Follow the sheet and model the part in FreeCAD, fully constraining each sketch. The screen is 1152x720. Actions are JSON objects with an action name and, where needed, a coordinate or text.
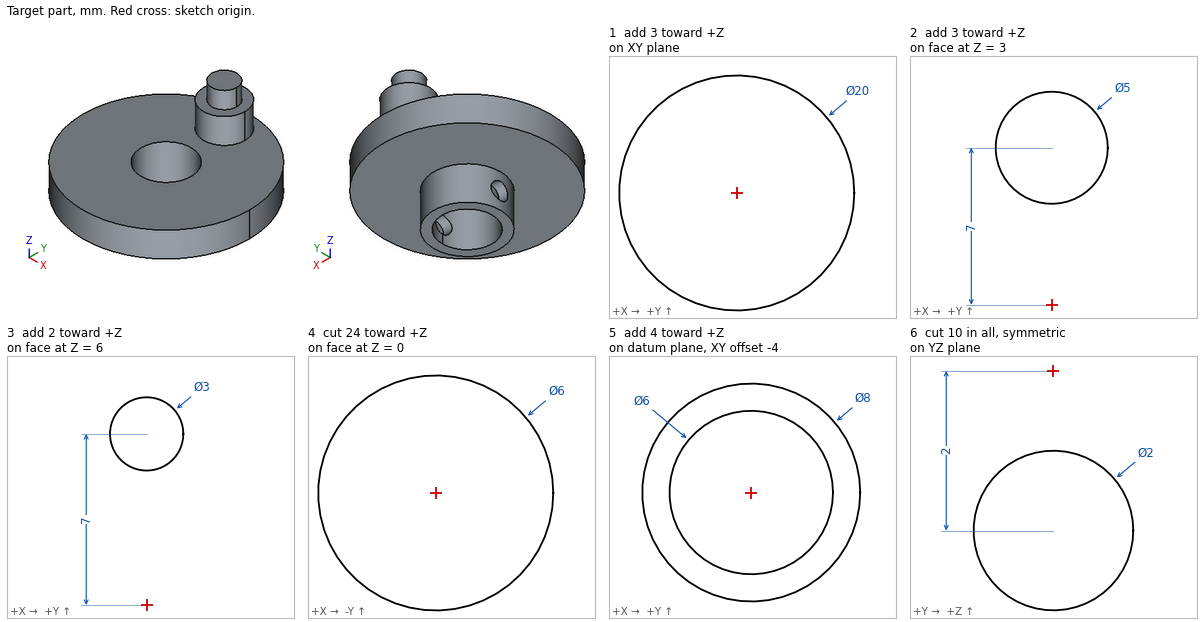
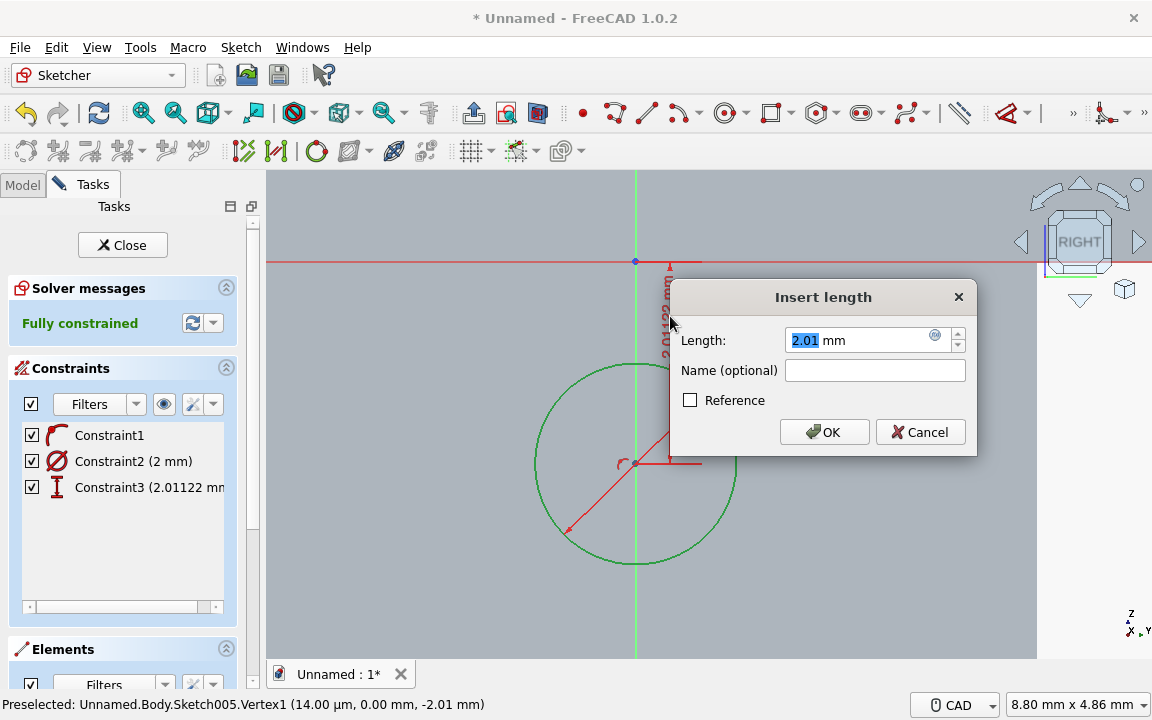
{"action": "type", "text": "2"}
{"action": "key", "text": "Return"}
{"action": "key", "text": "Escape"}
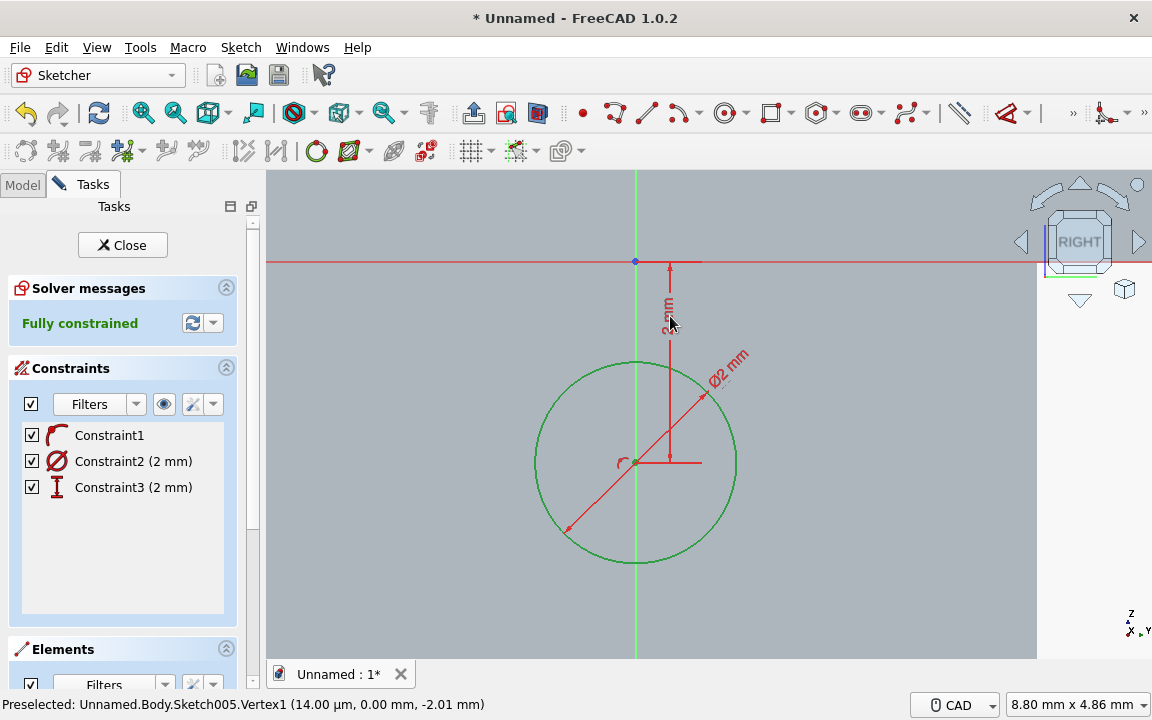
{"action": "left_click", "coordinate": [123, 245]}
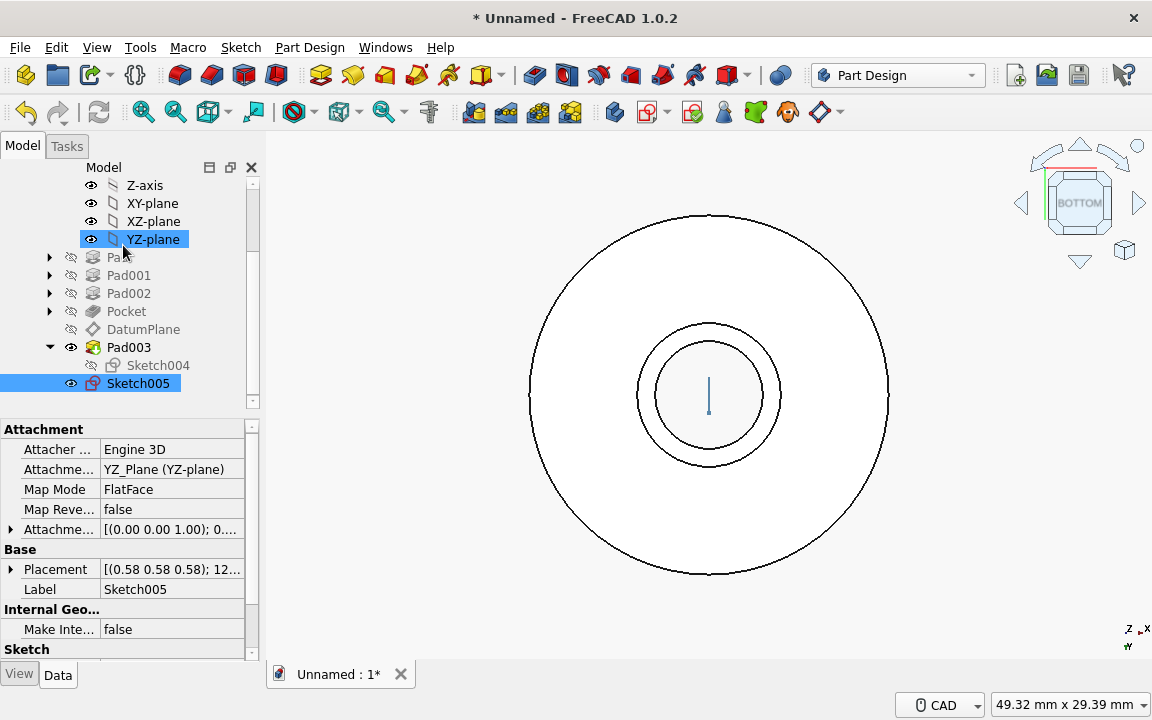
{"action": "left_click", "coordinate": [536, 76]}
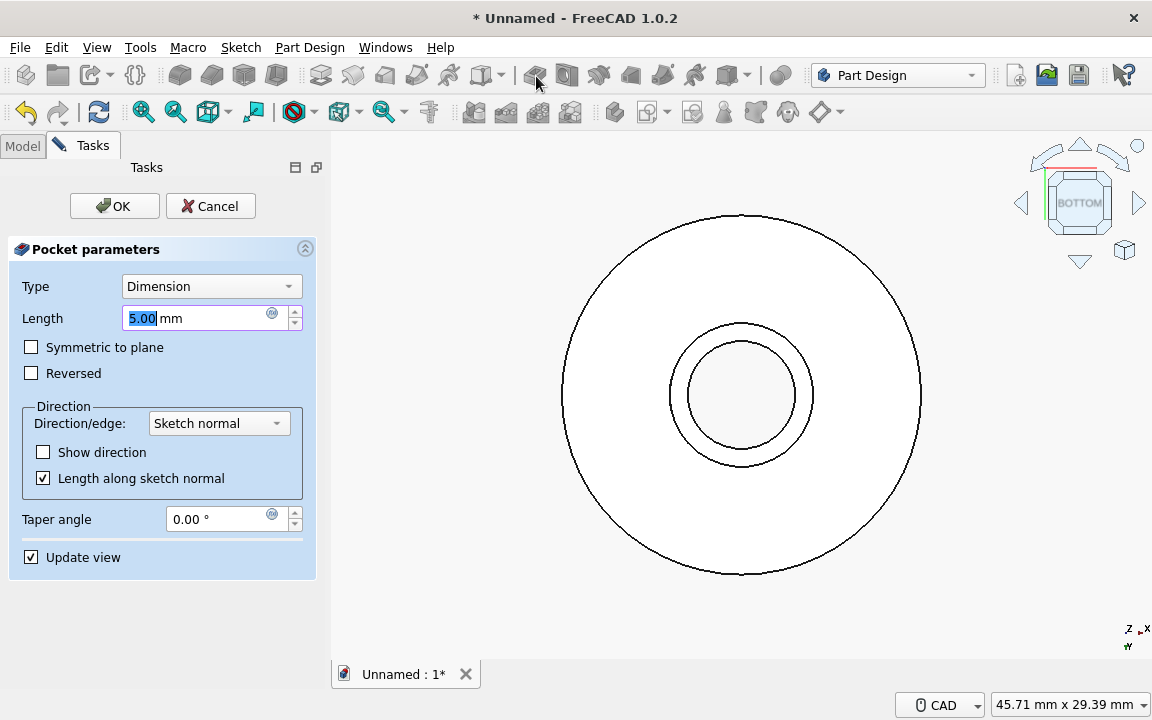
{"action": "type", "text": "10"}
{"action": "key", "text": "Tab"}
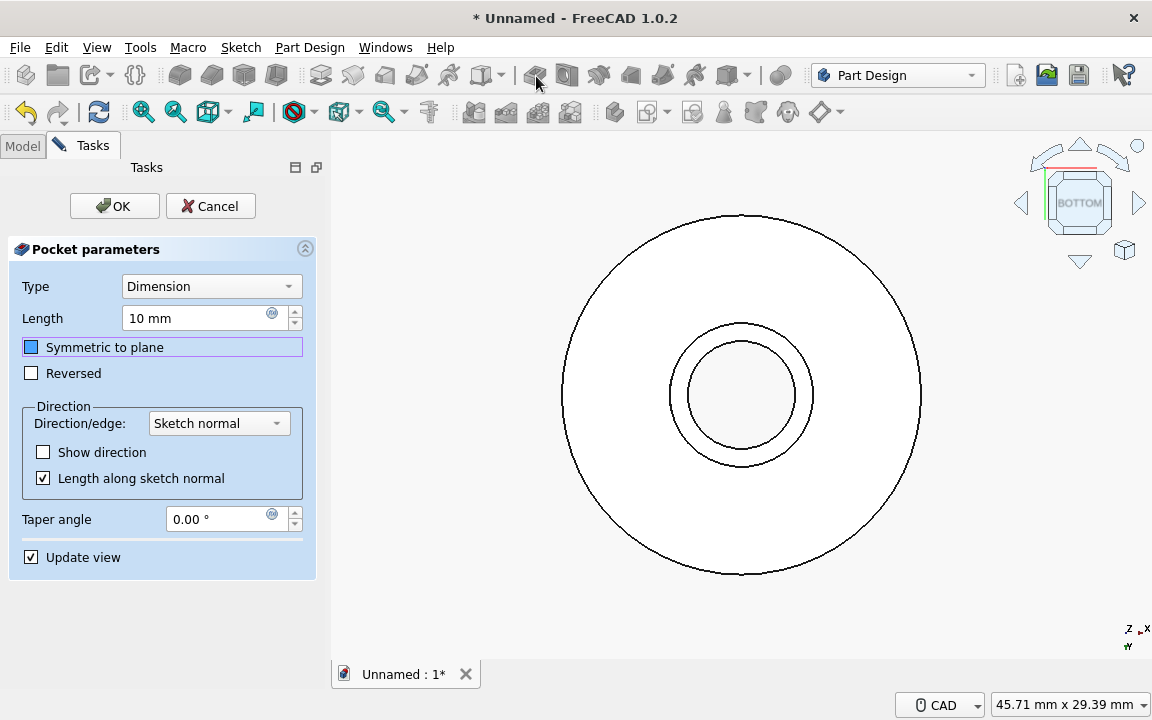
{"action": "left_click", "coordinate": [30, 347]}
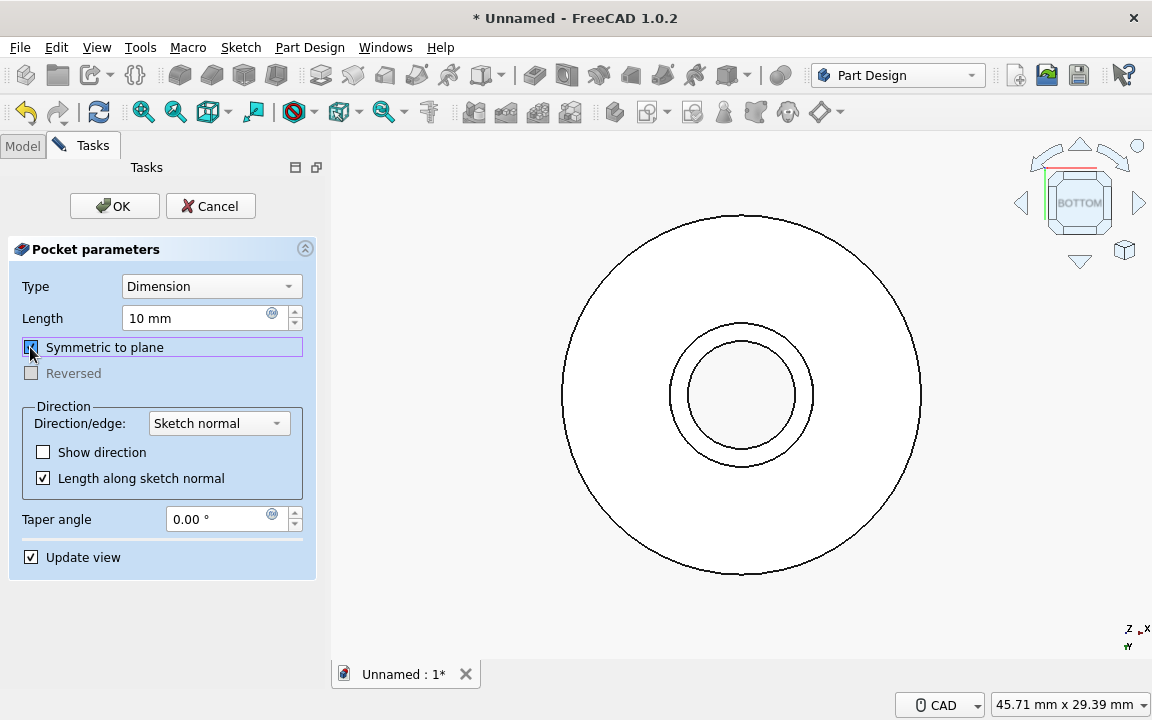
{"action": "left_click", "coordinate": [115, 206]}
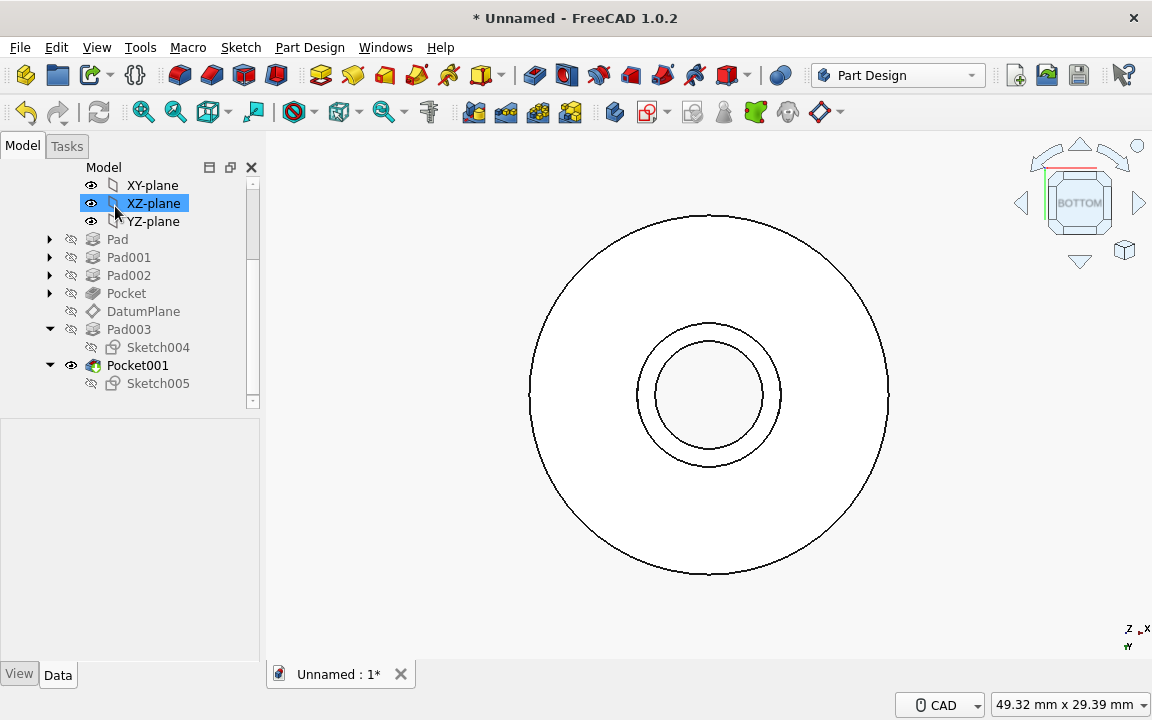
{"action": "key", "text": "0"}